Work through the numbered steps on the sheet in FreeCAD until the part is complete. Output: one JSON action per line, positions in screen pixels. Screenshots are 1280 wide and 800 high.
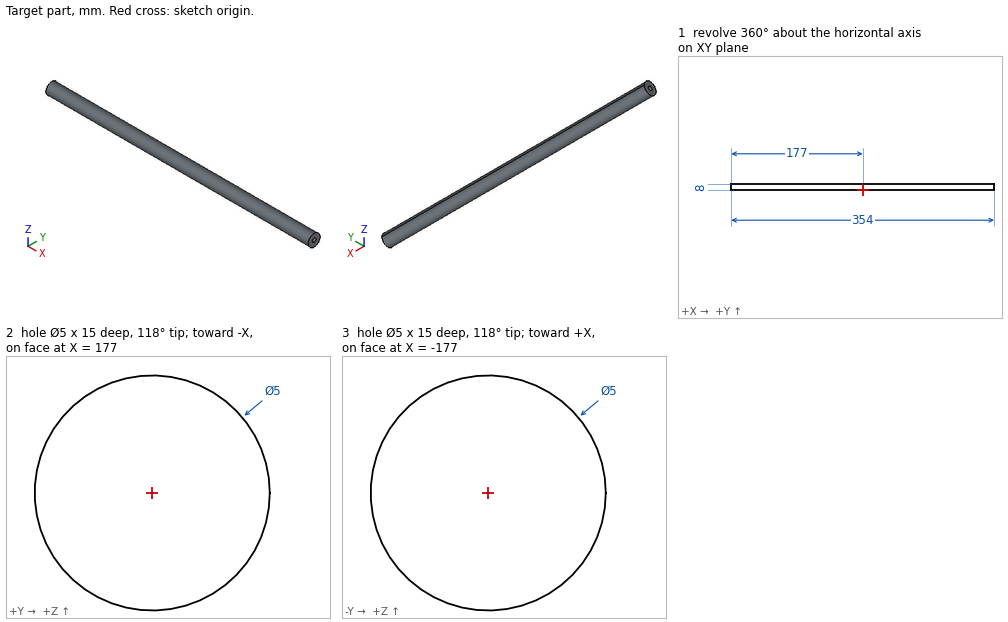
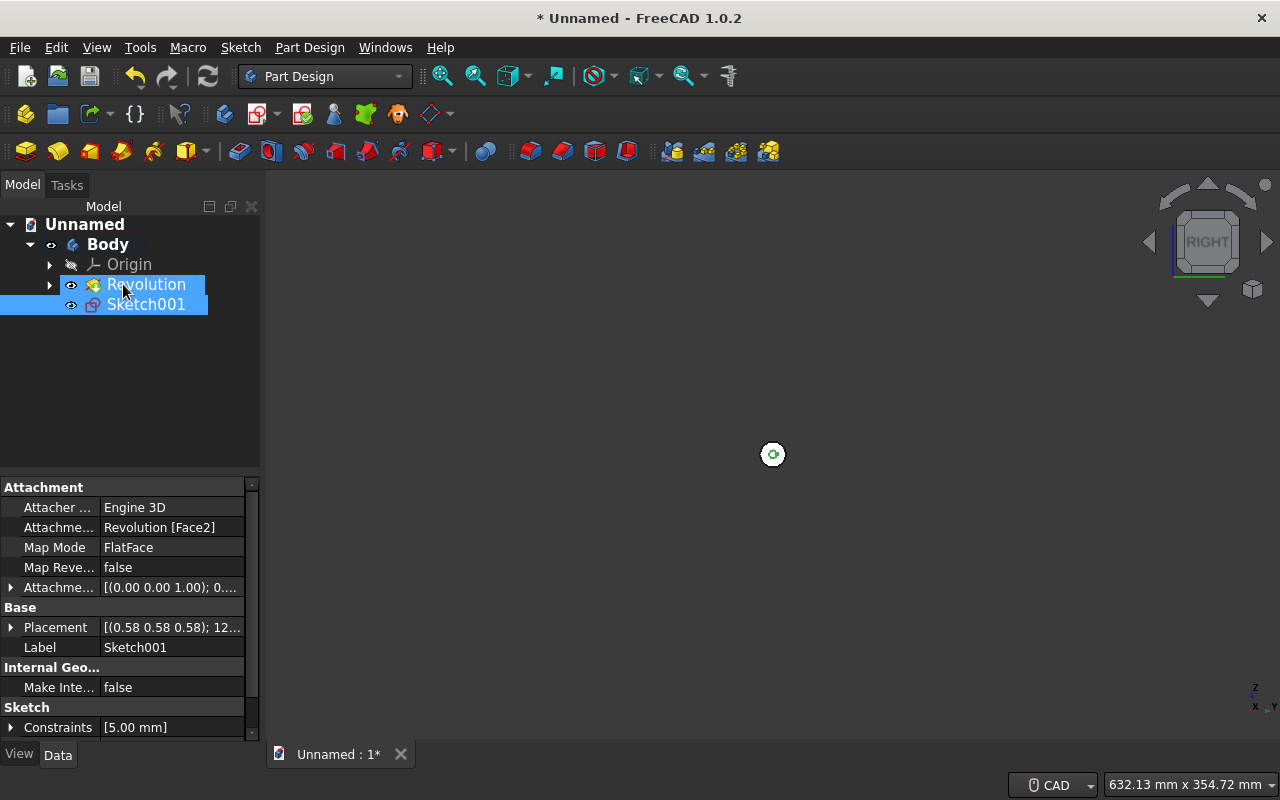
{"action": "left_click", "coordinate": [272, 152]}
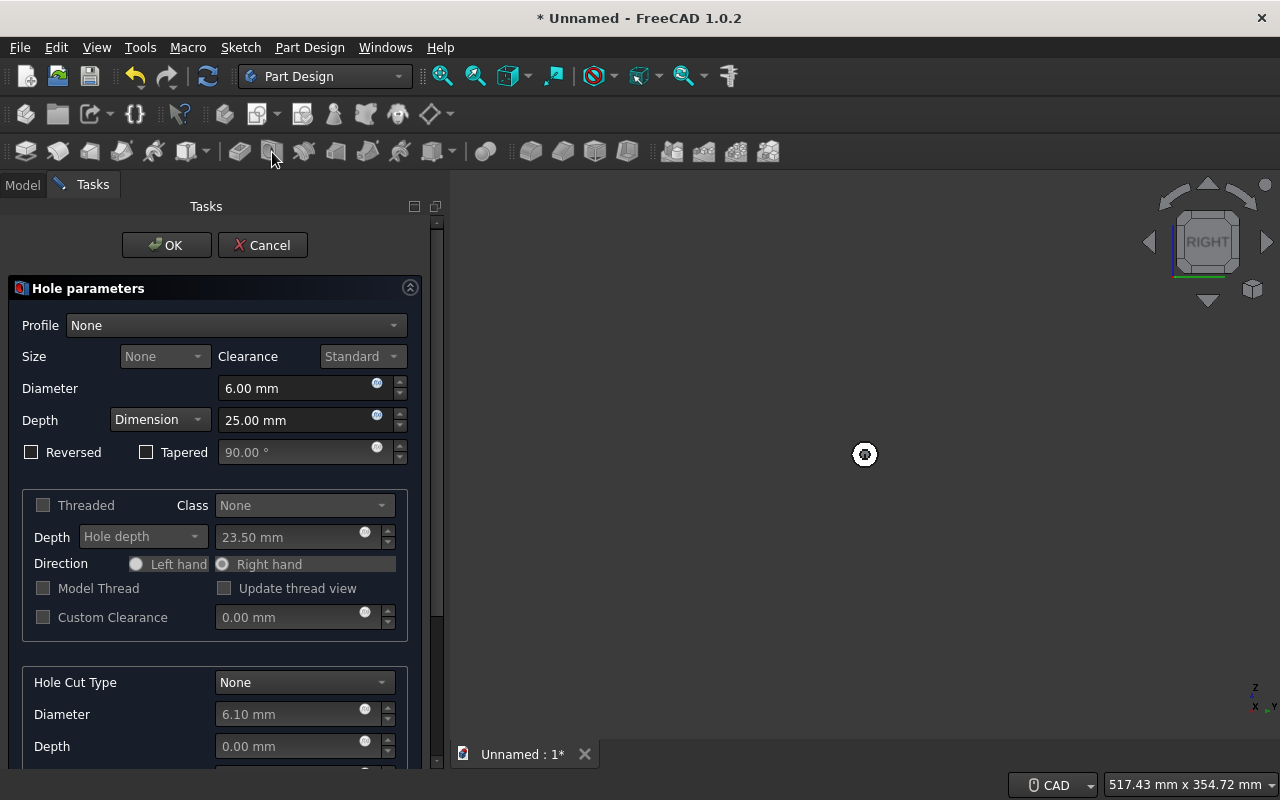
{"action": "triple_click", "coordinate": [305, 388]}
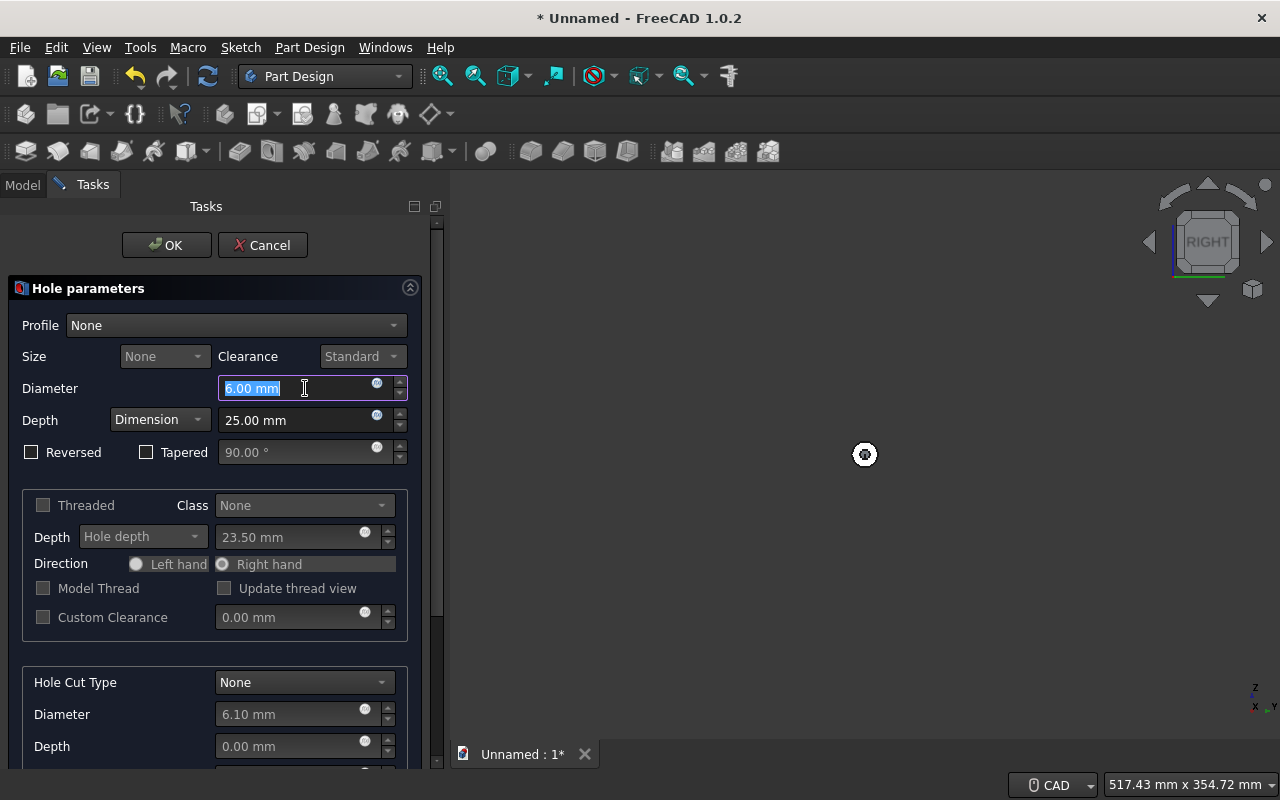
{"action": "type", "text": "5"}
{"action": "key", "text": "Tab"}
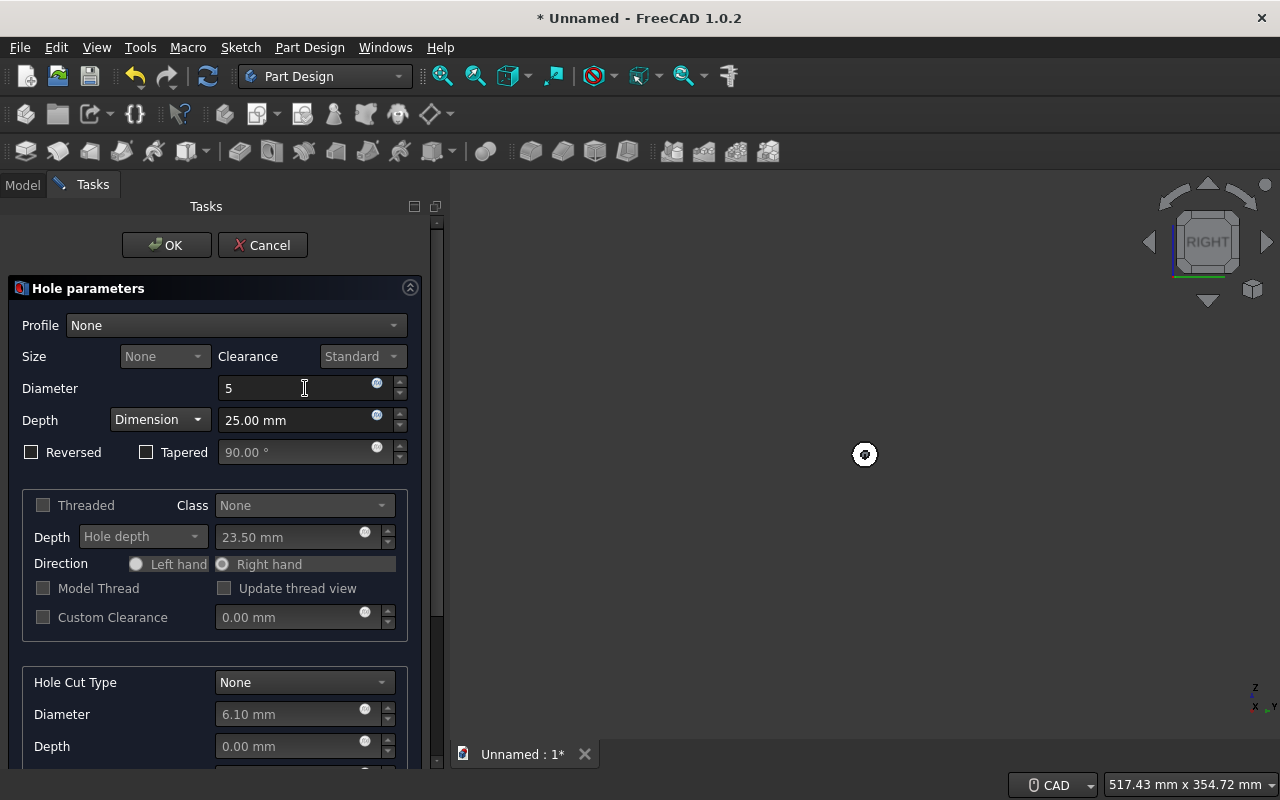
{"action": "triple_click", "coordinate": [305, 420]}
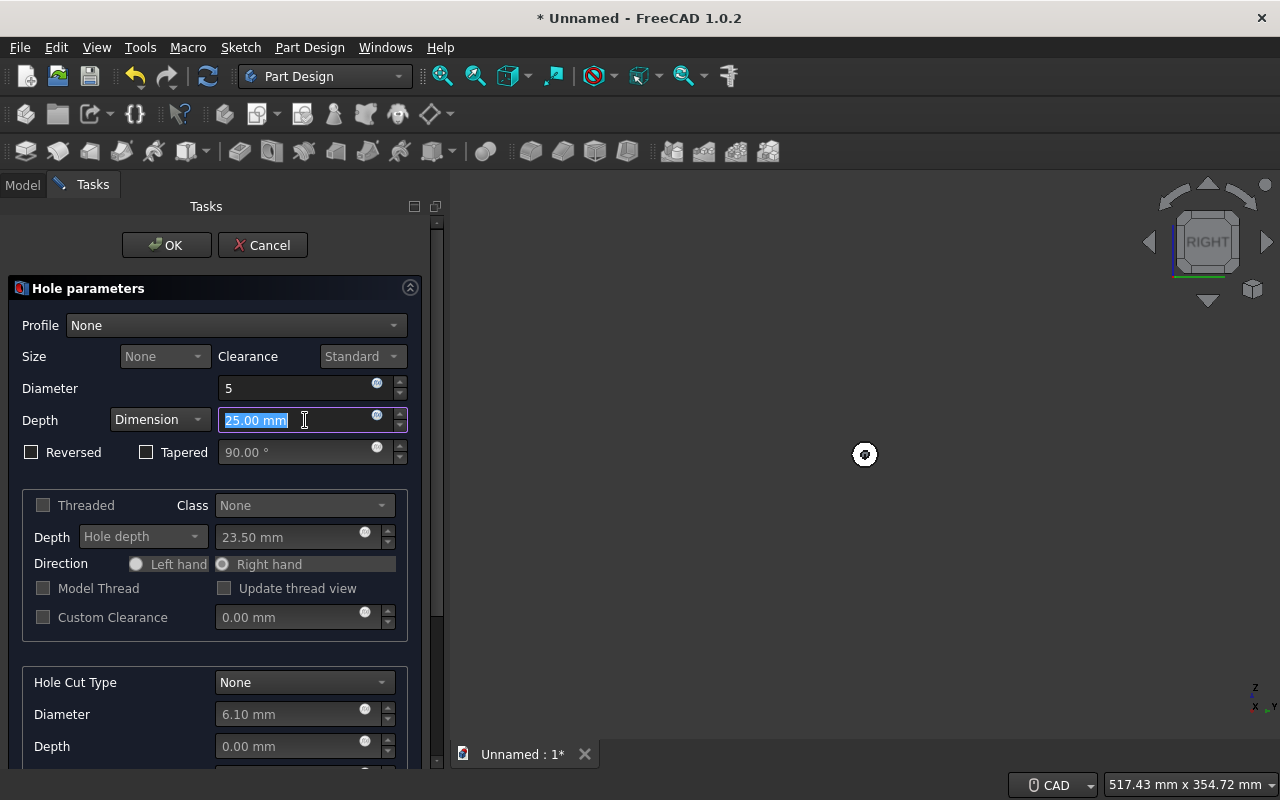
{"action": "type", "text": "15"}
{"action": "key", "text": "Tab"}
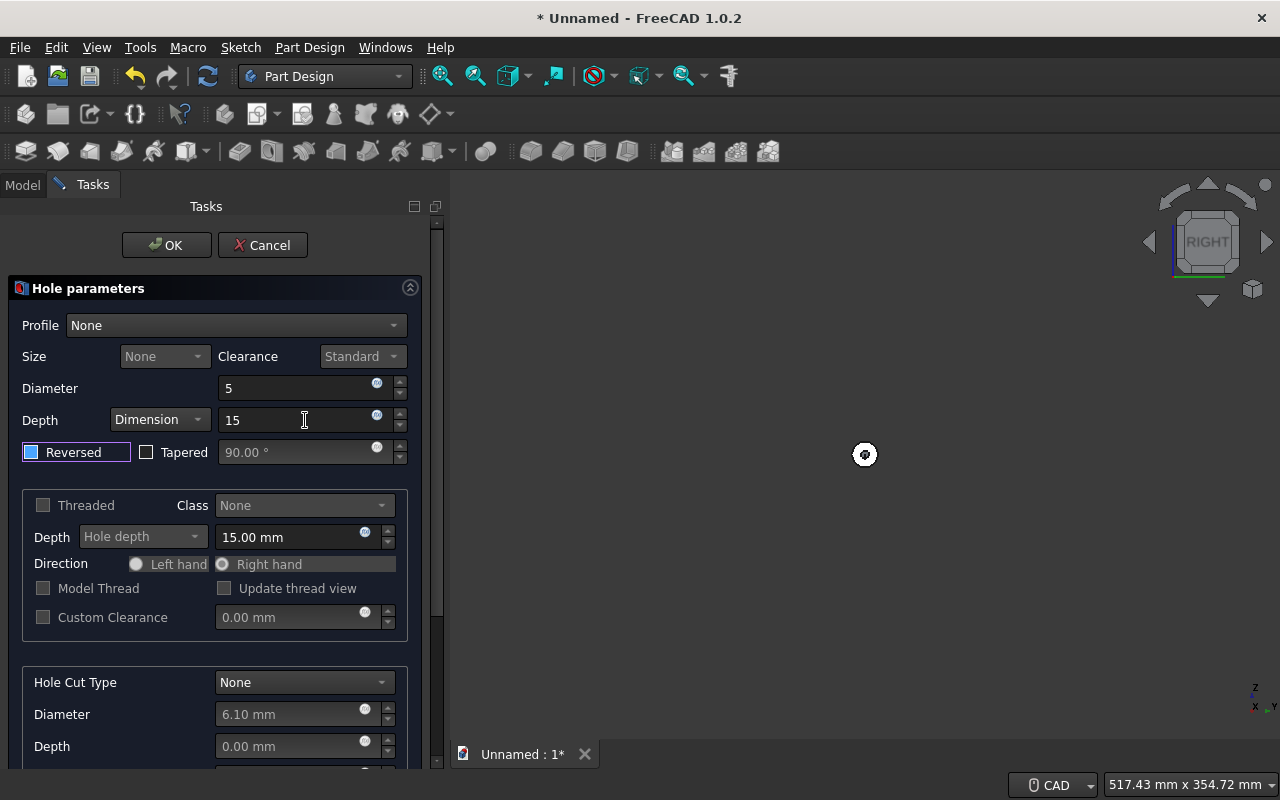
{"action": "left_click", "coordinate": [167, 245]}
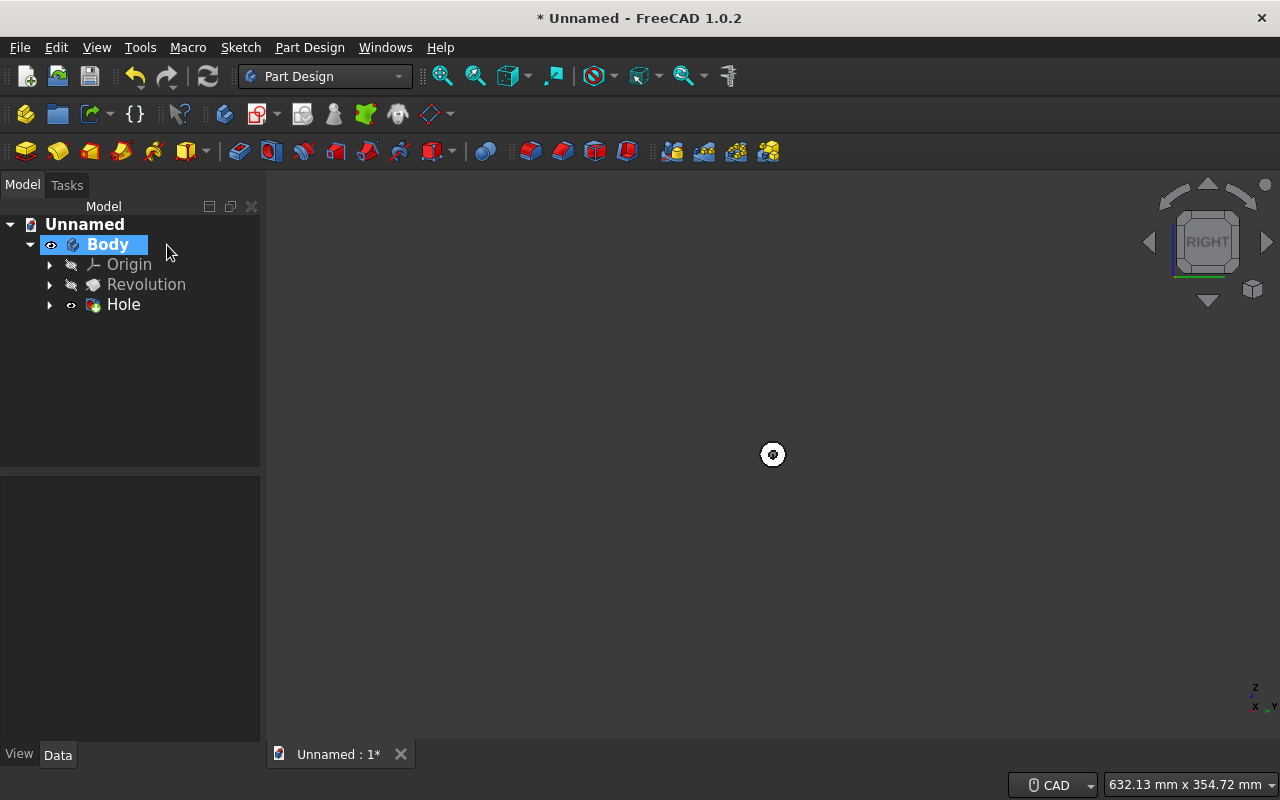
{"action": "left_click", "coordinate": [444, 76]}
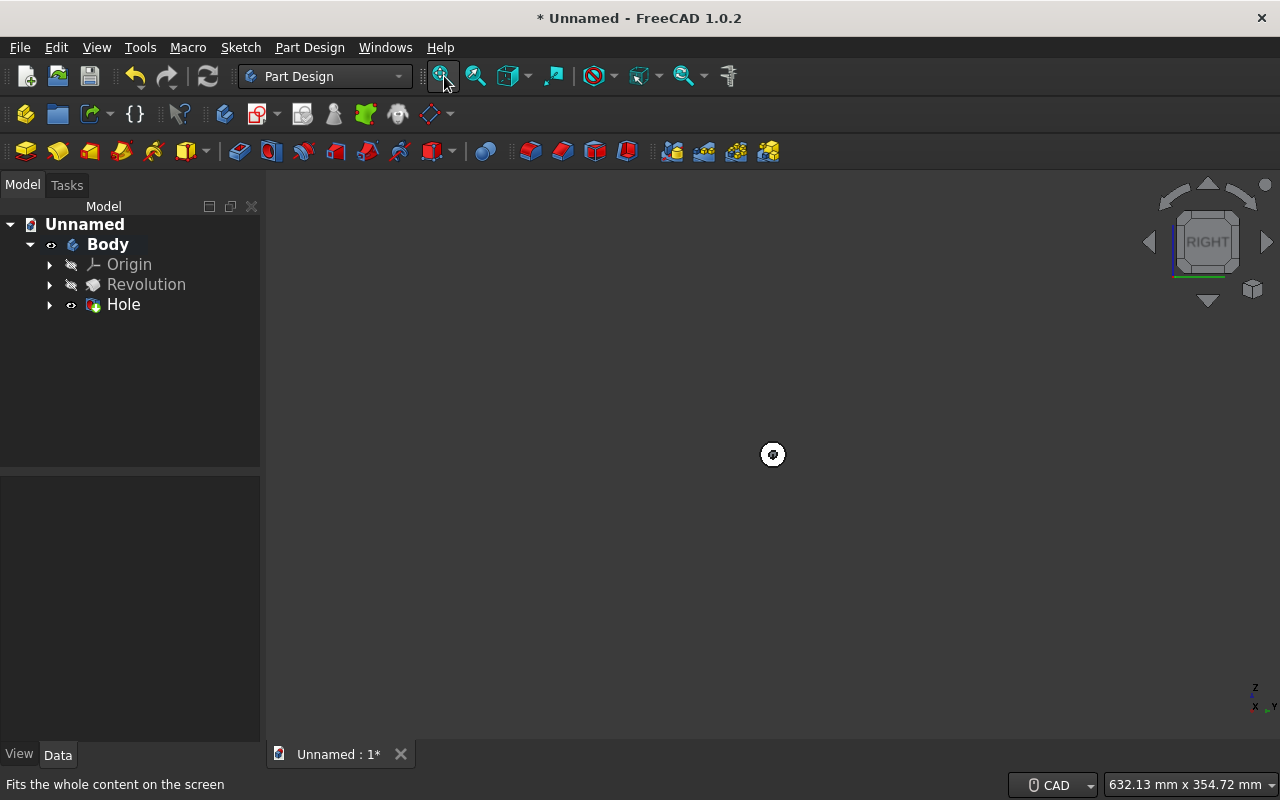
{"action": "key", "text": "6"}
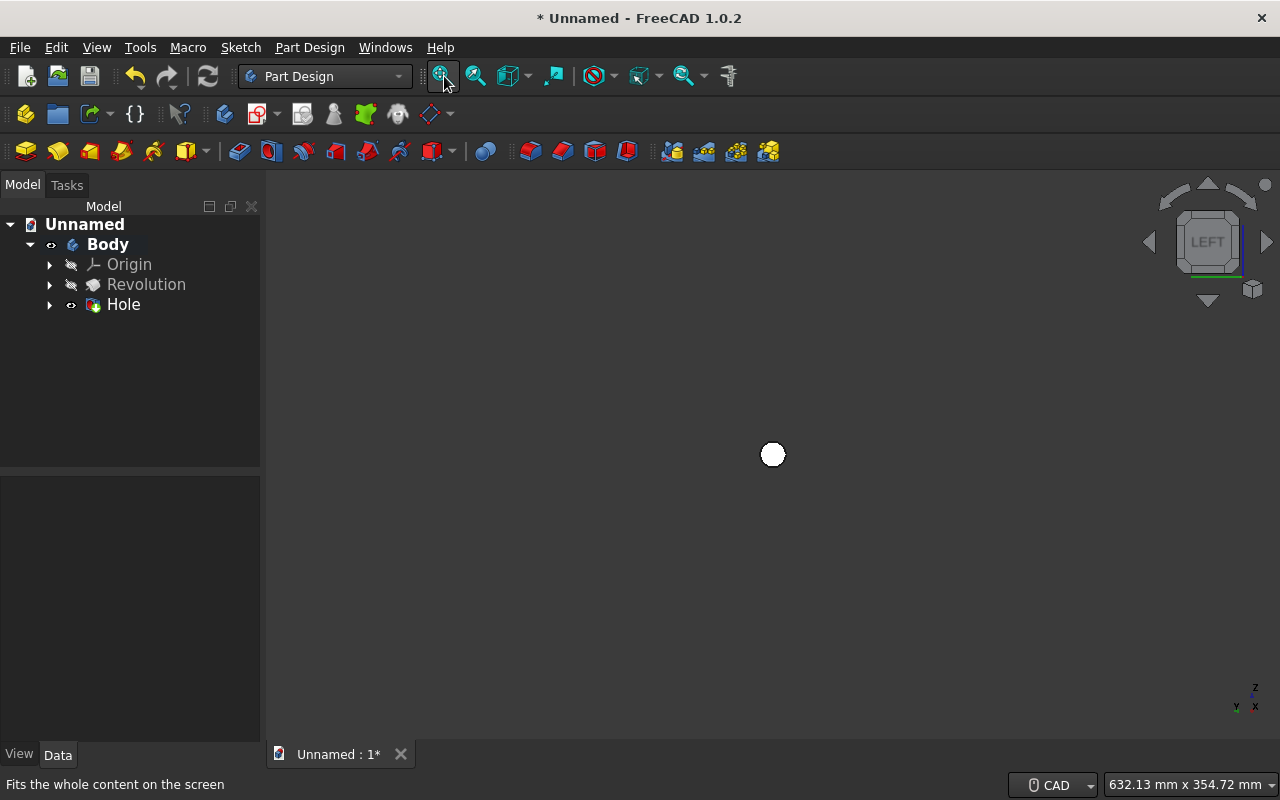
{"action": "left_click", "coordinate": [444, 76]}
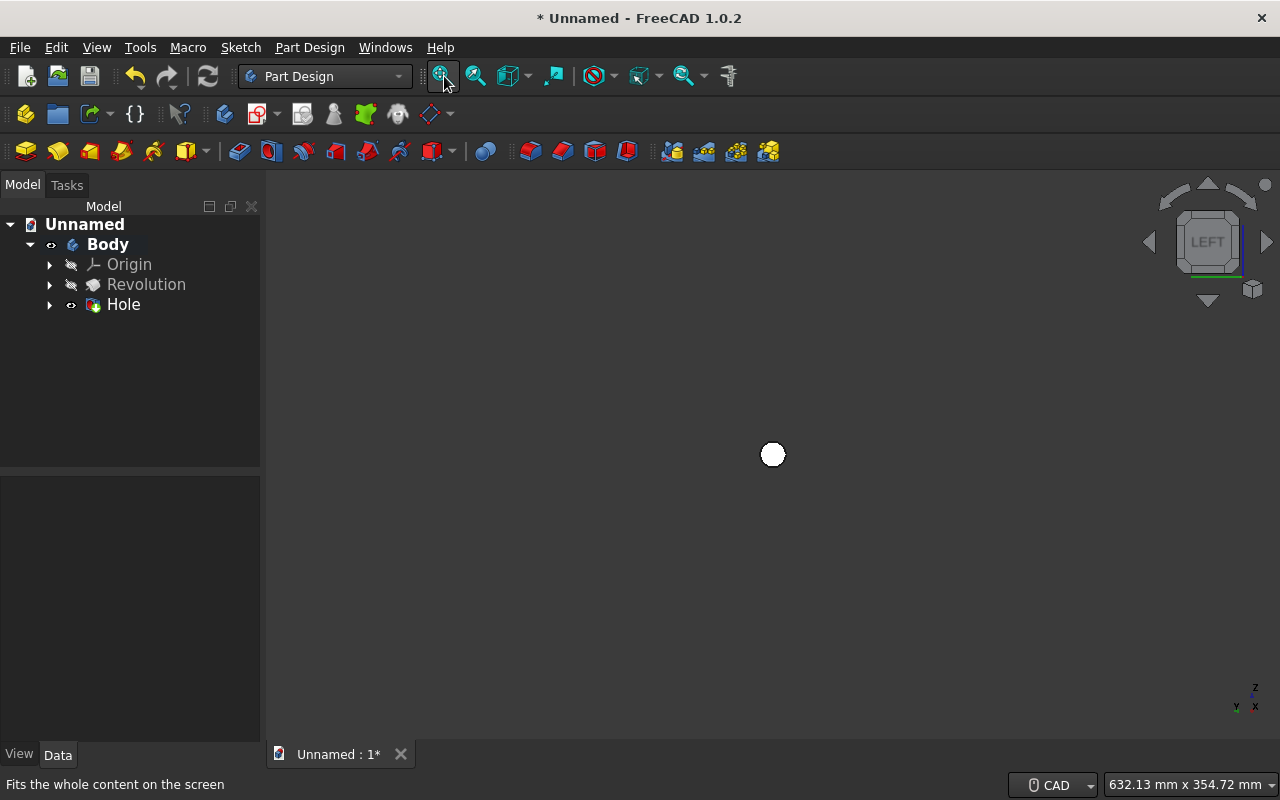
{"action": "left_click", "coordinate": [773, 453]}